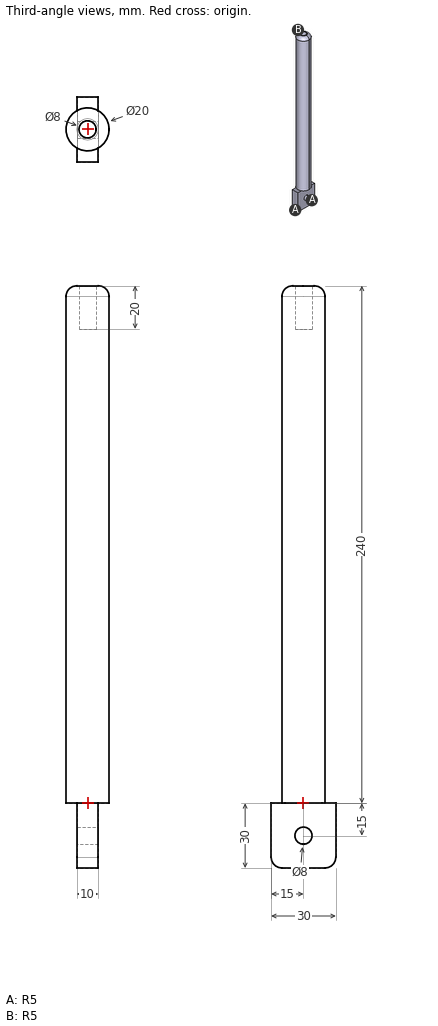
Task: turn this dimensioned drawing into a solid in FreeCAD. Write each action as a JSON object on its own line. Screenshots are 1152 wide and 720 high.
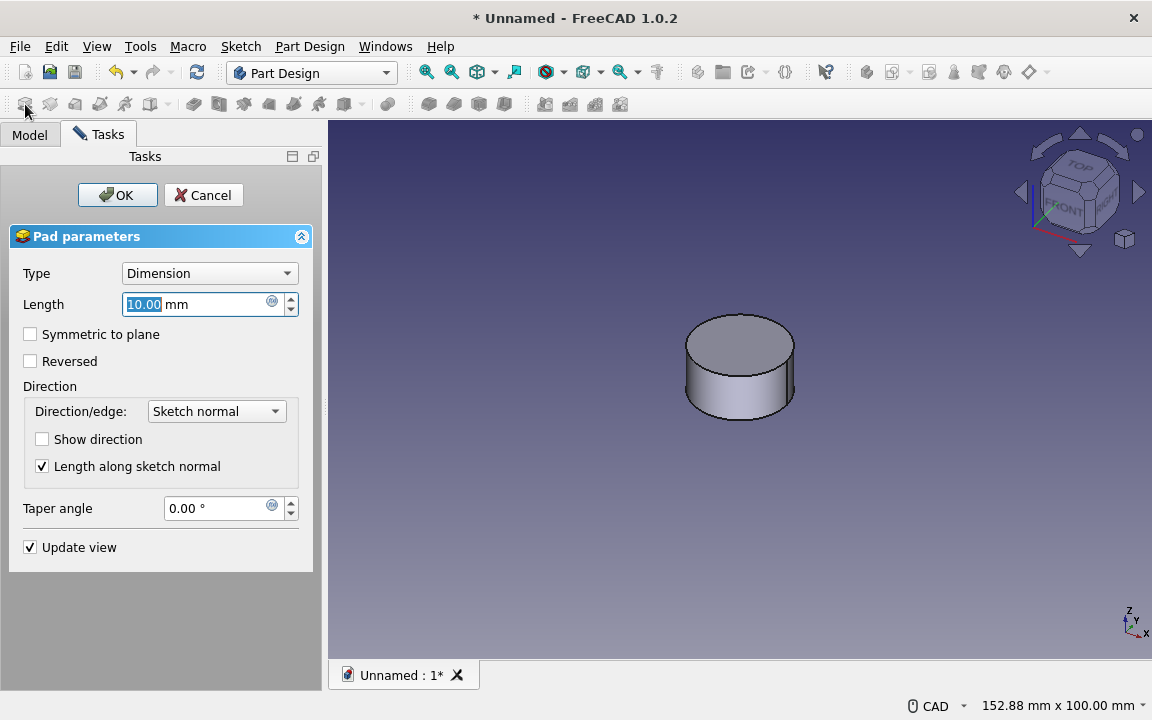
{"action": "type", "text": "240"}
{"action": "key", "text": "Tab"}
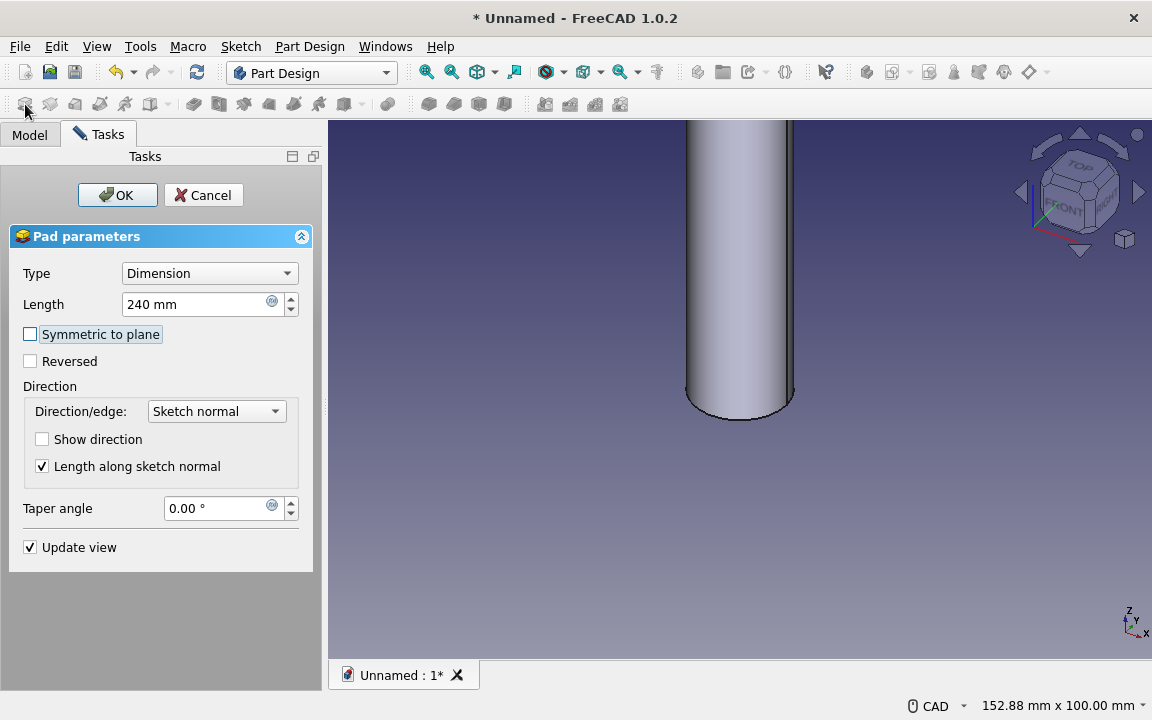
{"action": "left_click", "coordinate": [118, 195]}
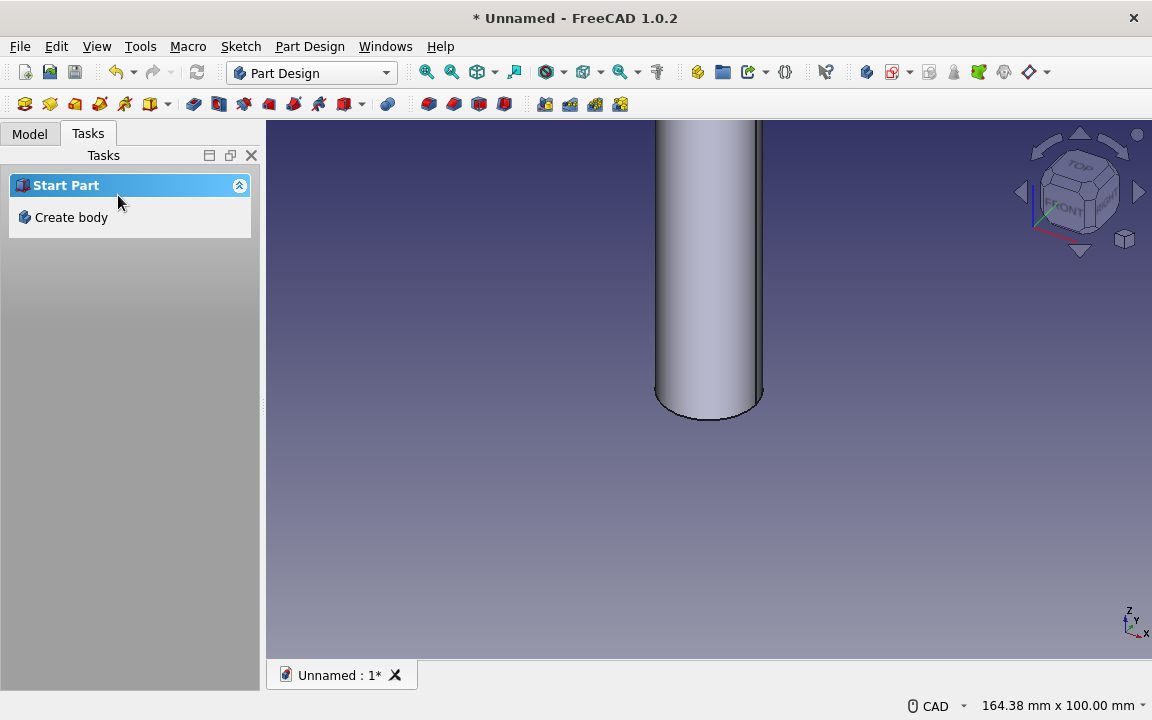
{"action": "key", "text": "v f"}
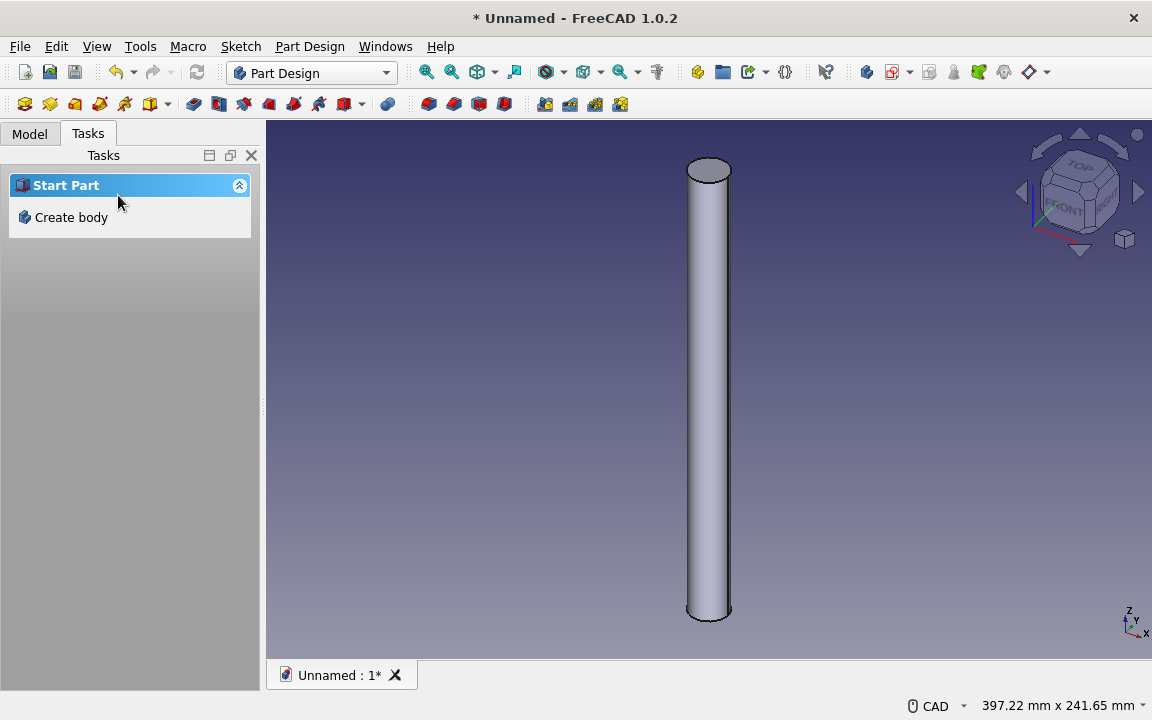
{"action": "left_click", "coordinate": [892, 72]}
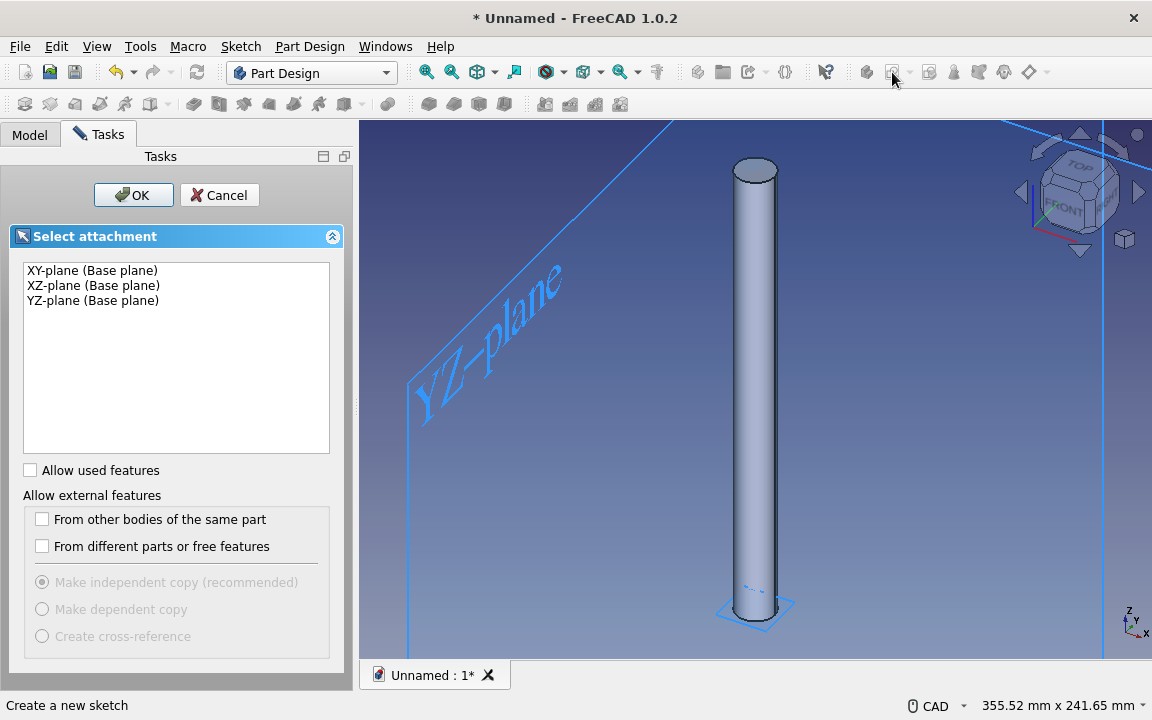
{"action": "left_click", "coordinate": [84, 300]}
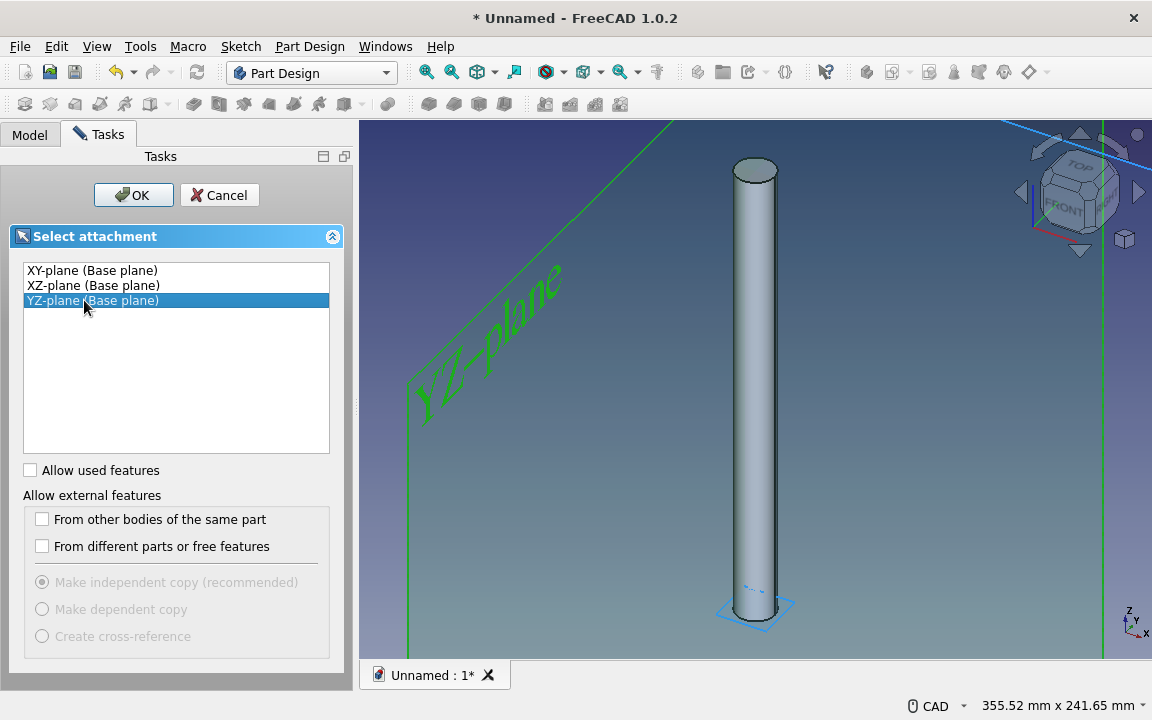
{"action": "left_click", "coordinate": [134, 195]}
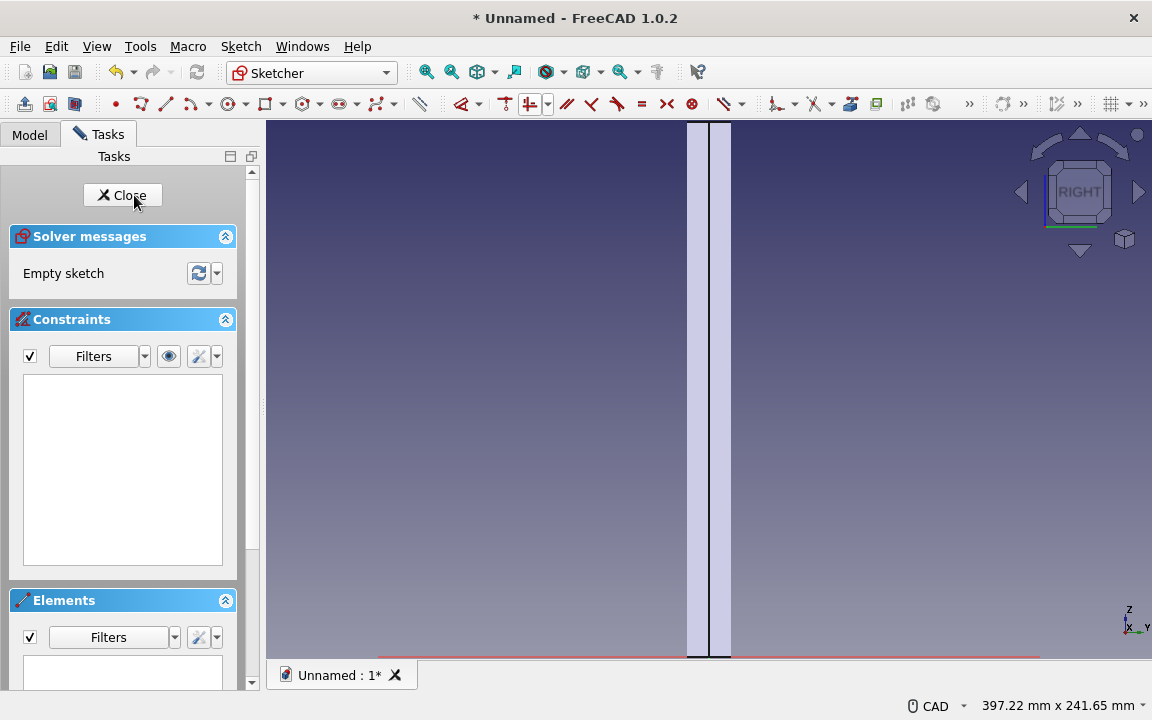
{"action": "key", "text": "q s"}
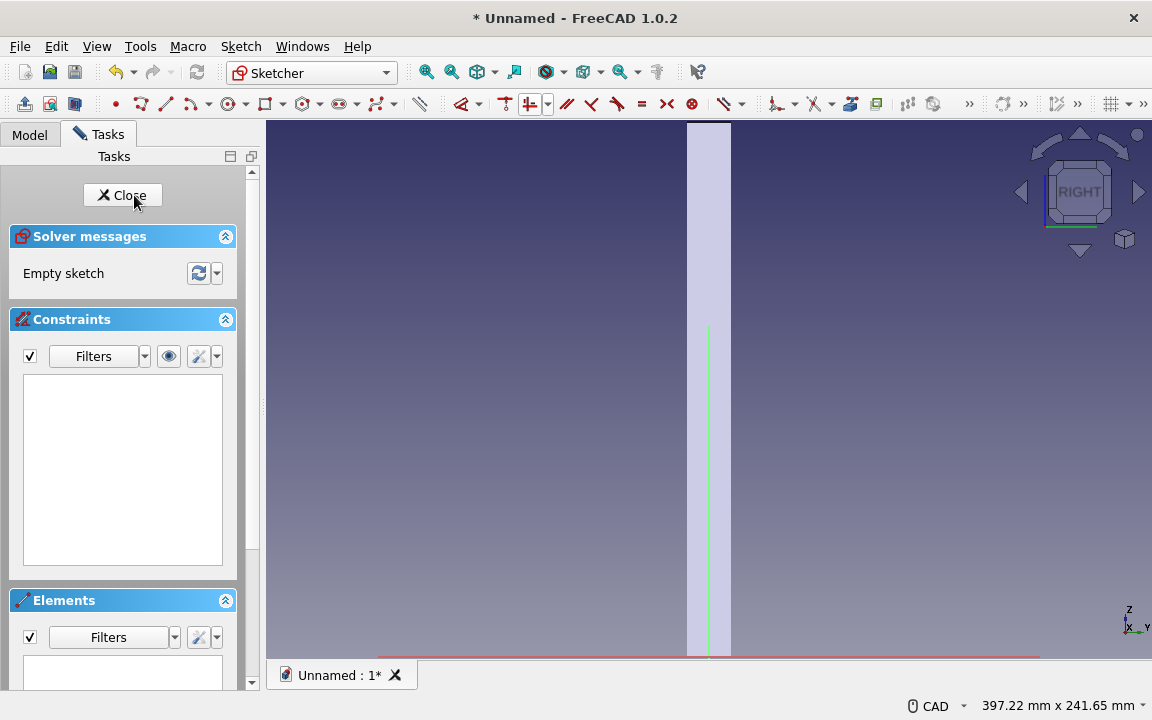
{"action": "scroll", "coordinate": [640, 390], "scroll_direction": "down", "scroll_amount": 5}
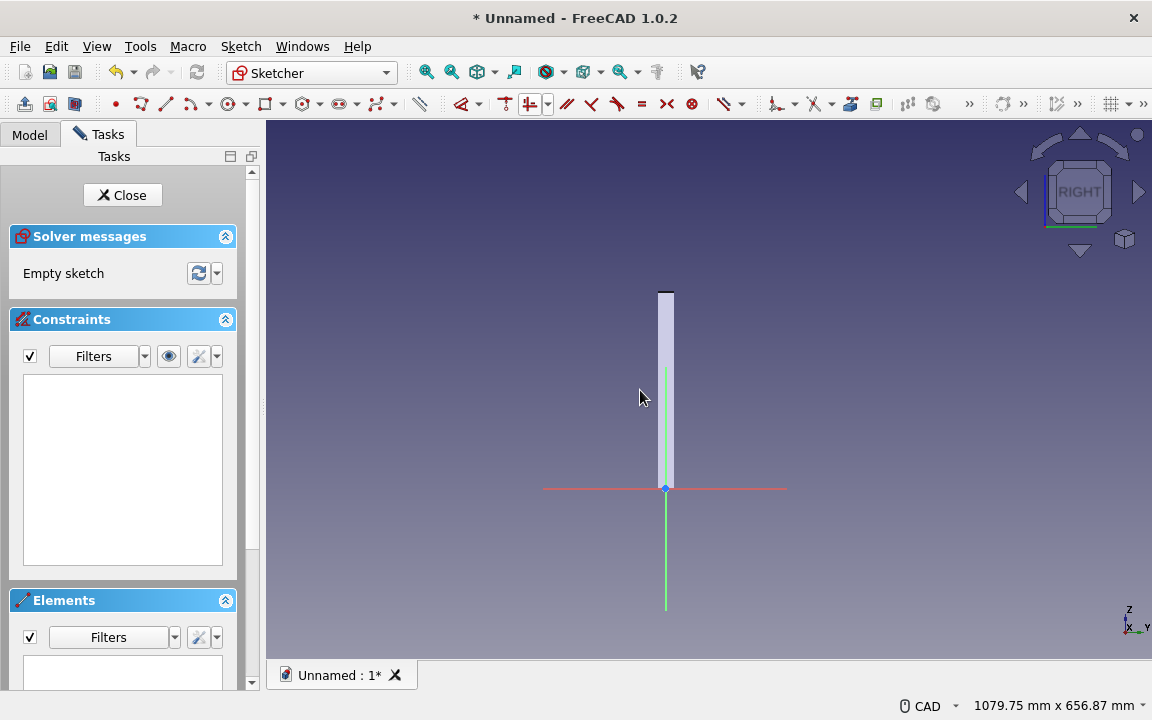
{"action": "scroll", "coordinate": [668, 510], "scroll_direction": "up", "scroll_amount": 13}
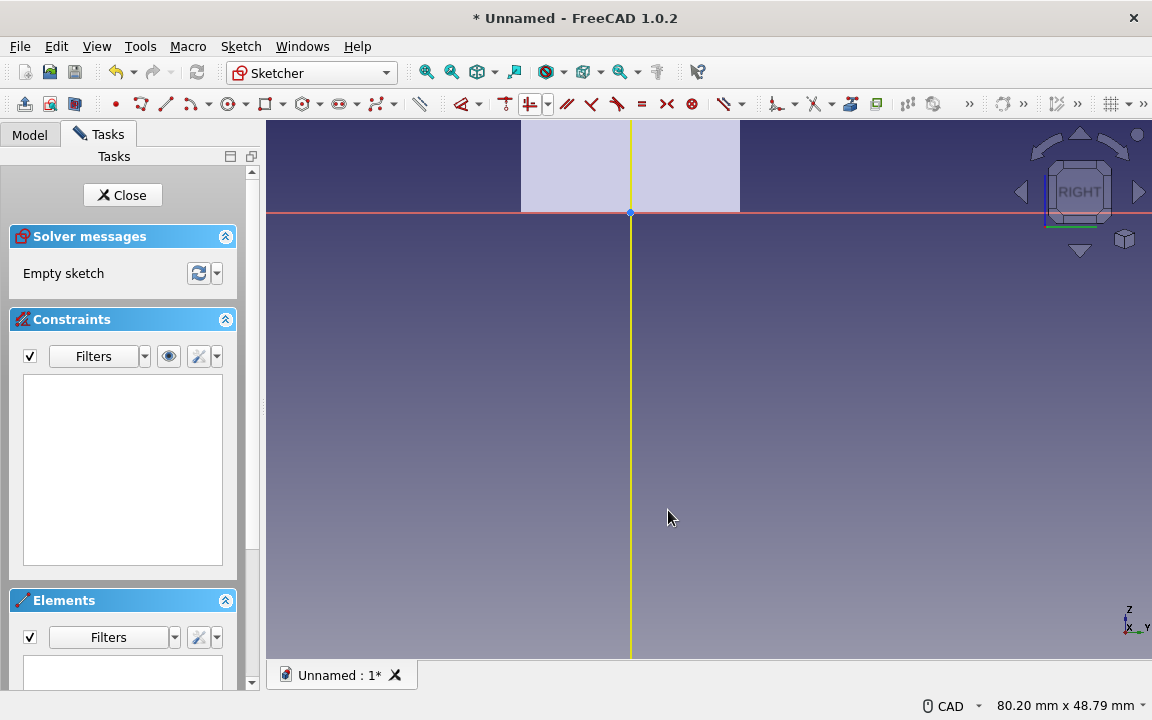
{"action": "key", "text": "g r"}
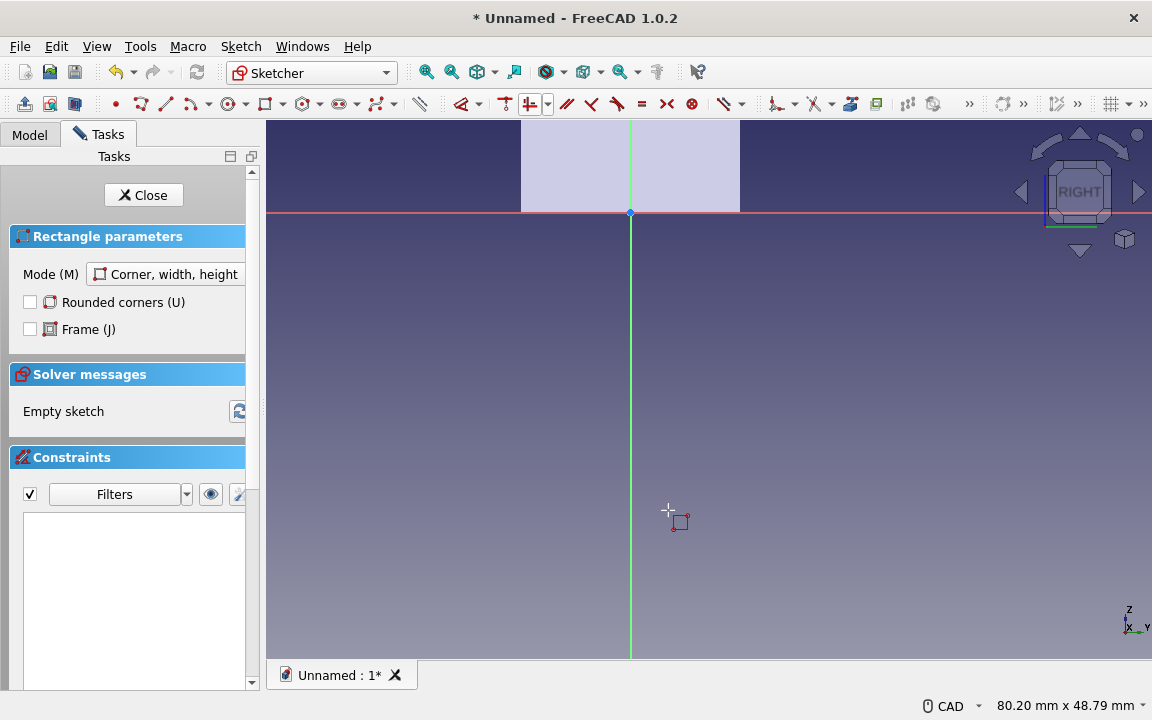
{"action": "left_click", "coordinate": [465, 213]}
{"action": "left_click", "coordinate": [796, 544]}
{"action": "key", "text": "Escape"}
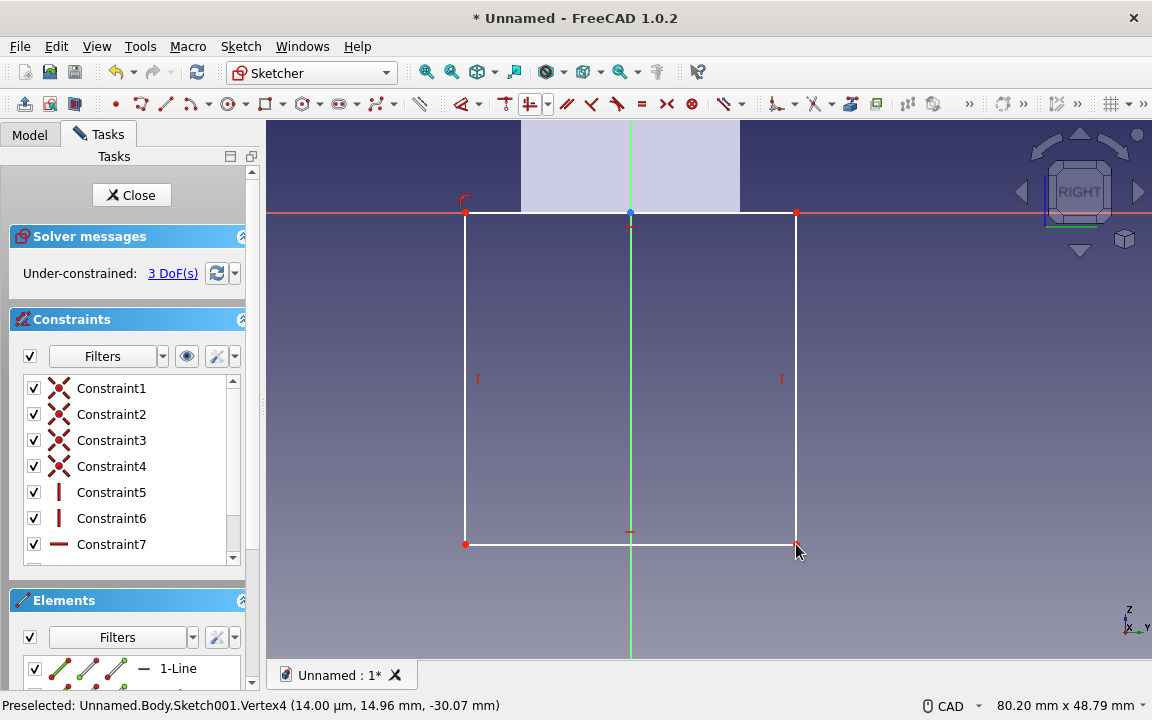
{"action": "left_click", "coordinate": [460, 104]}